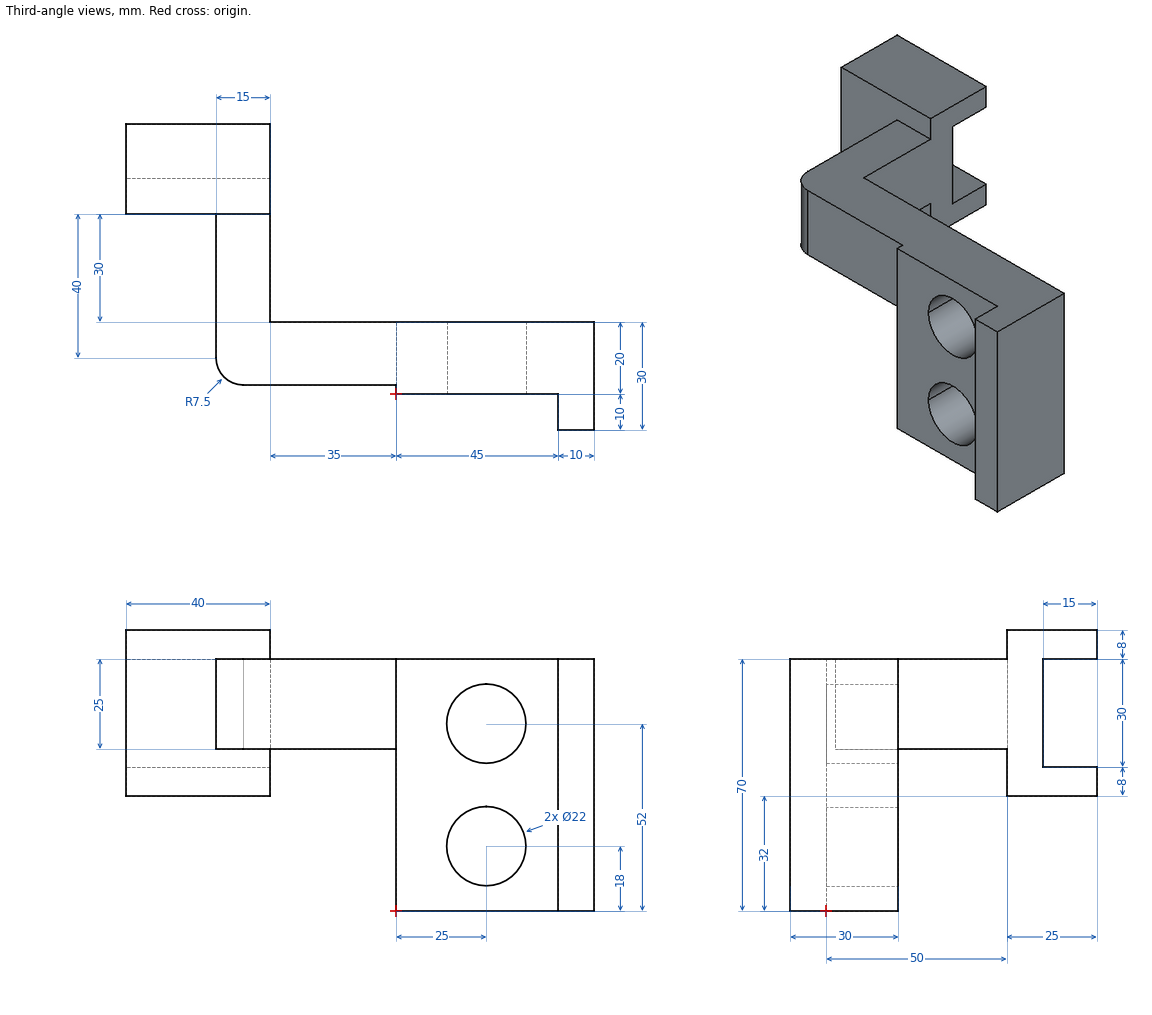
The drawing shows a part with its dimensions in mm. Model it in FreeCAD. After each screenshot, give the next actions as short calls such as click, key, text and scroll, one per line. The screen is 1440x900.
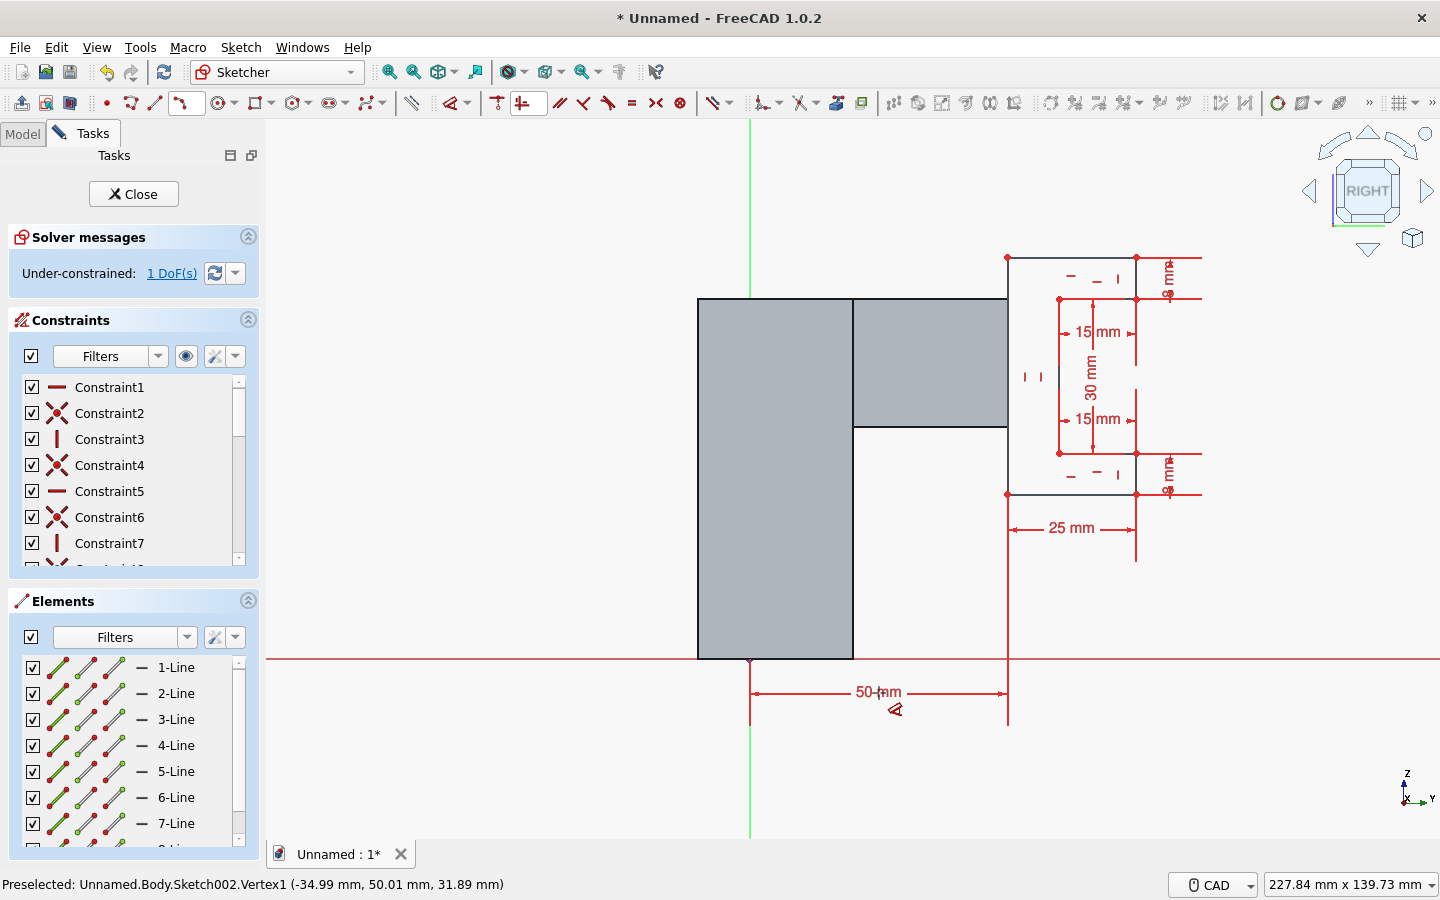
click(1008, 495)
click(716, 577)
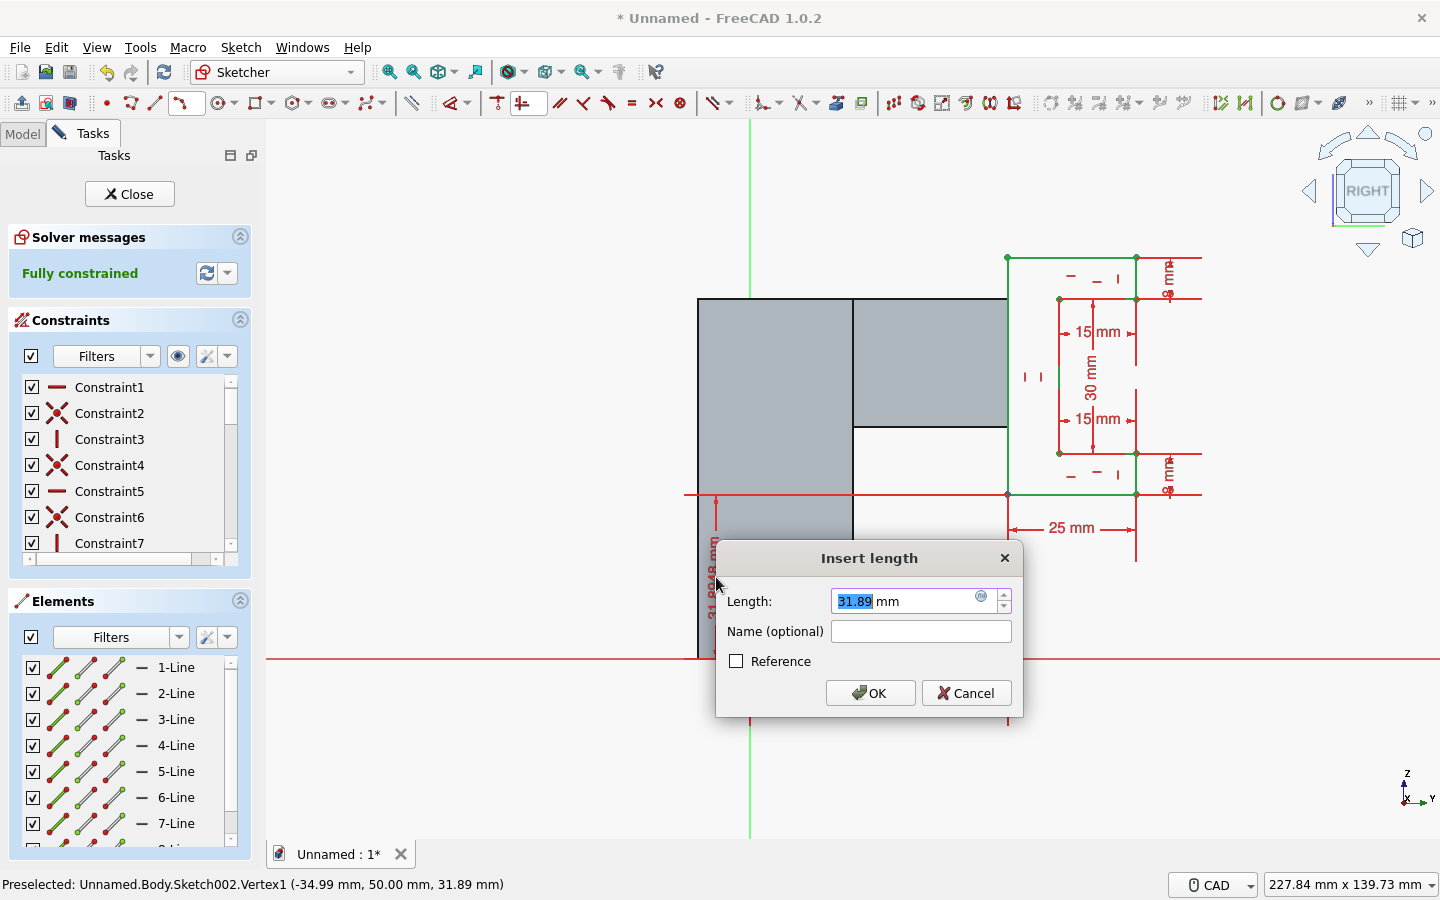
text(32)
key(Return)
key(Escape)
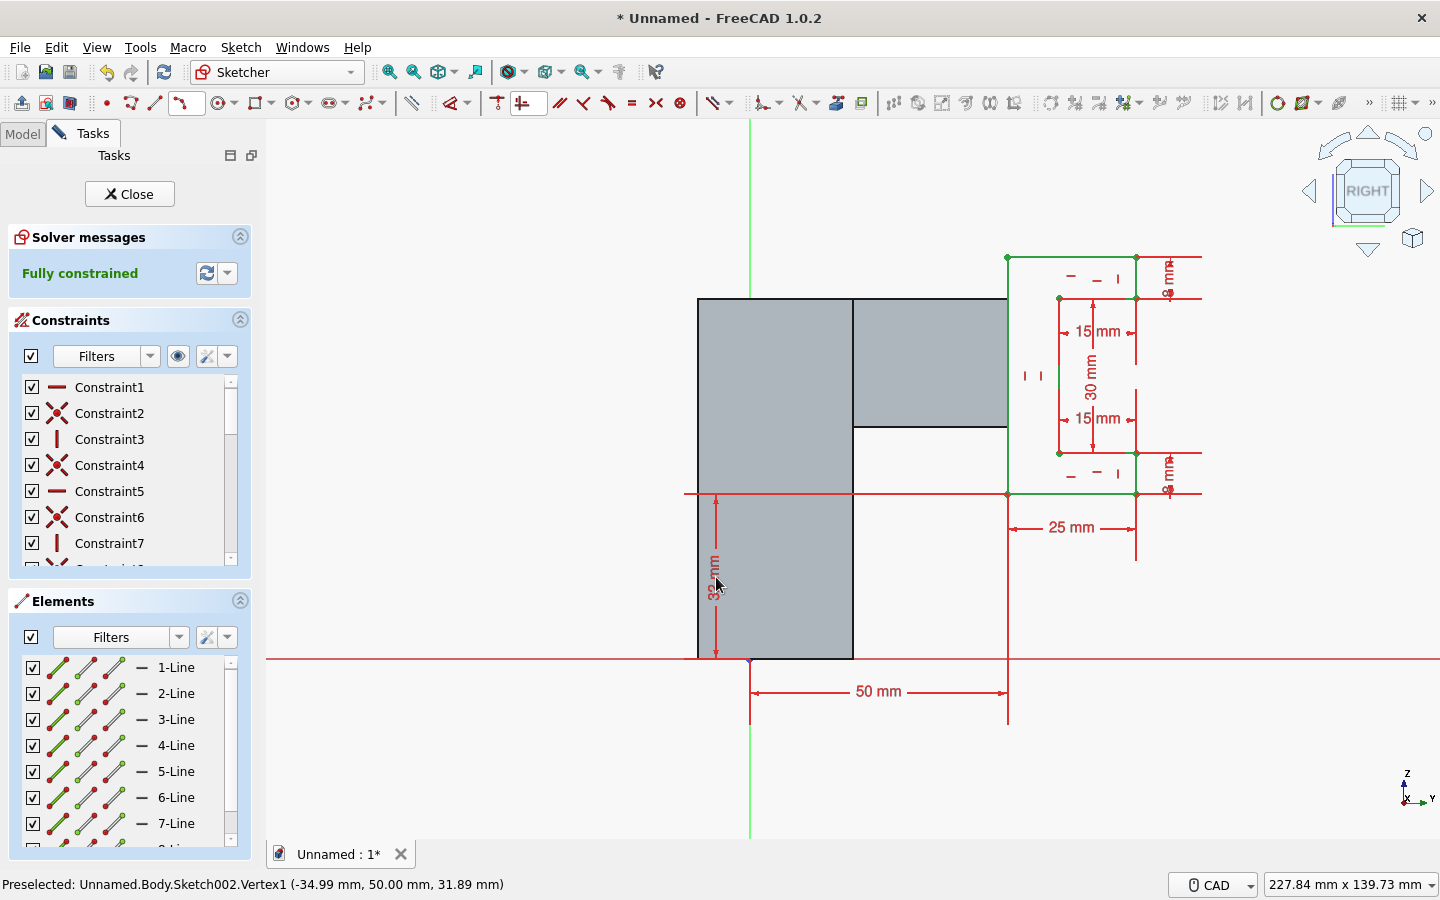
click(130, 194)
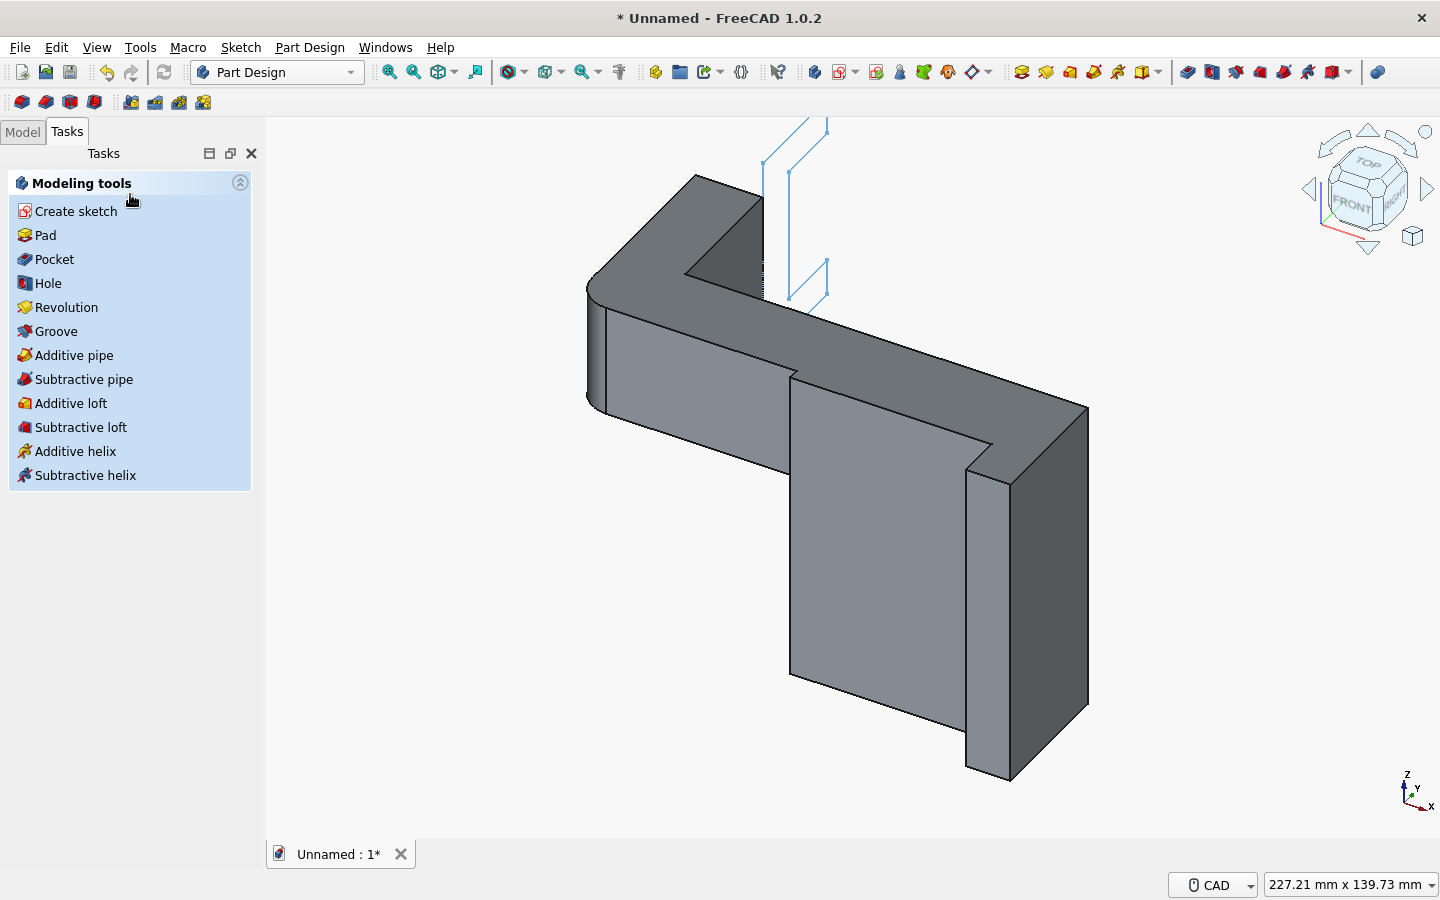
click(1022, 72)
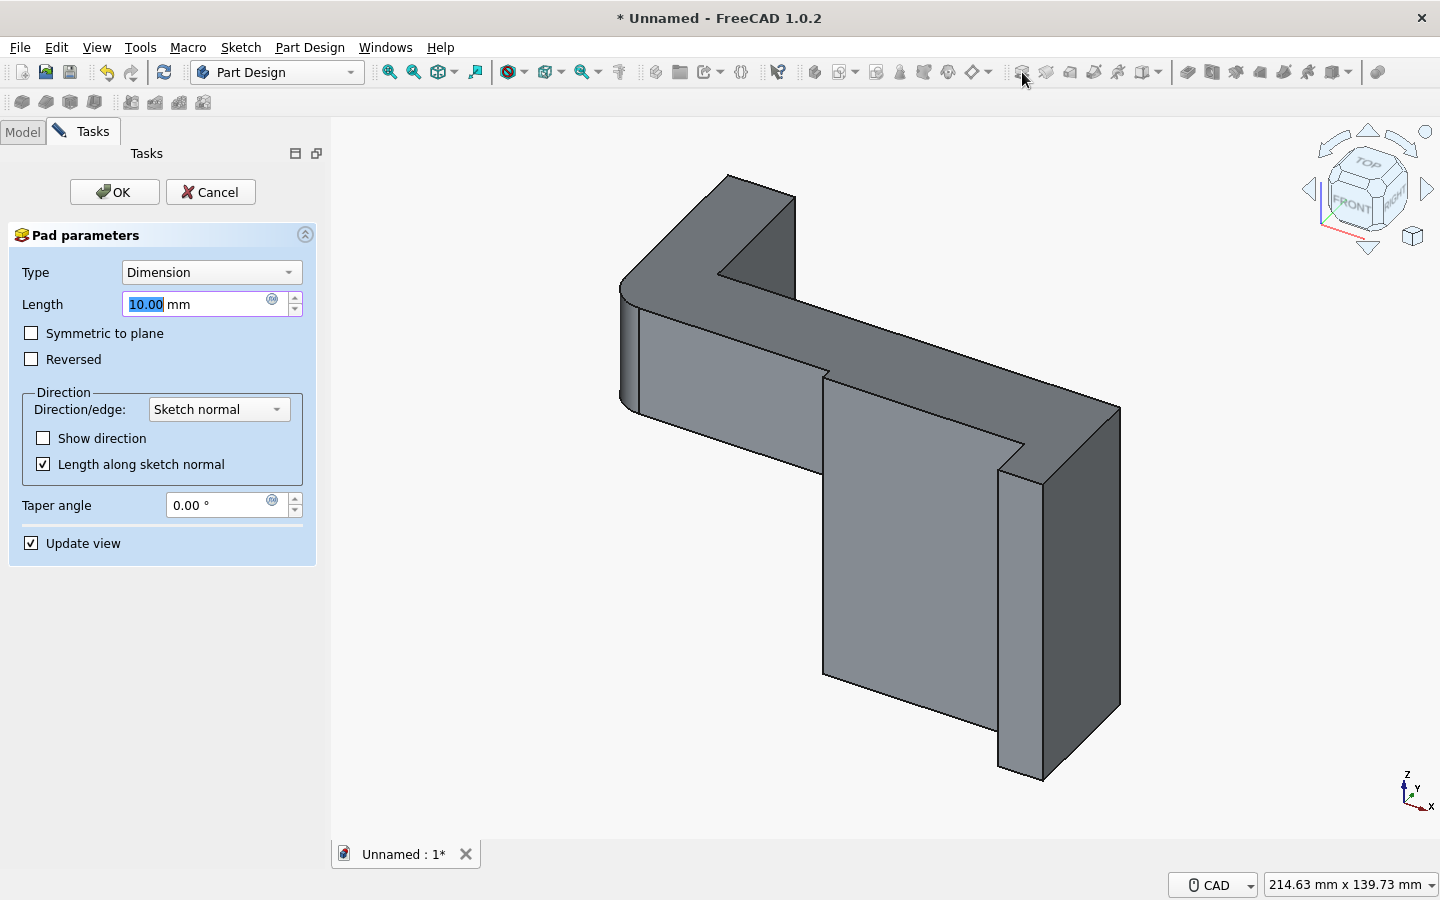
text(40)
key(Tab)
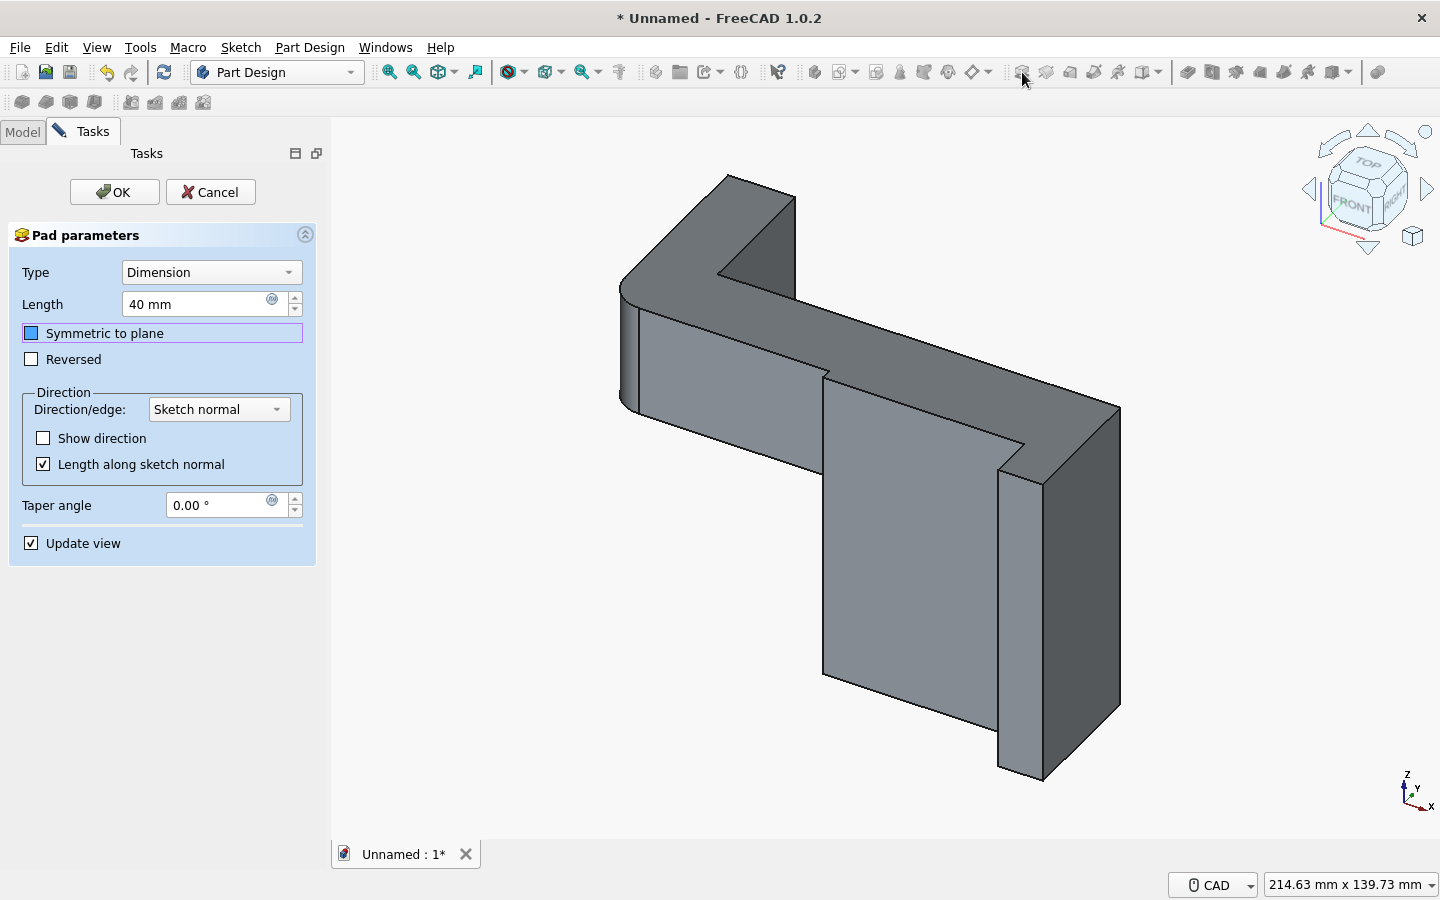
click(30, 359)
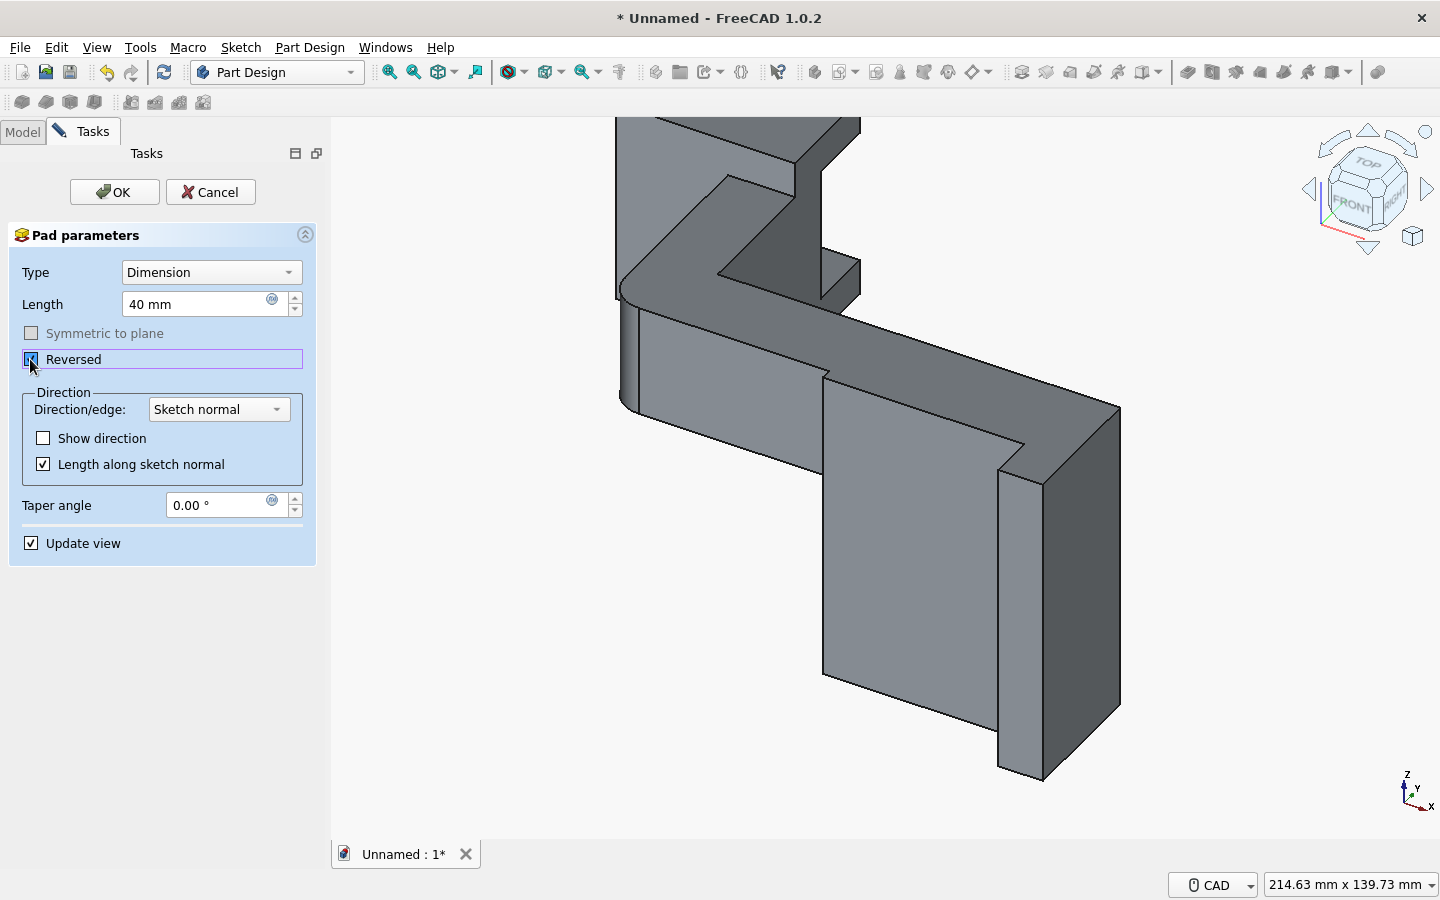
click(115, 192)